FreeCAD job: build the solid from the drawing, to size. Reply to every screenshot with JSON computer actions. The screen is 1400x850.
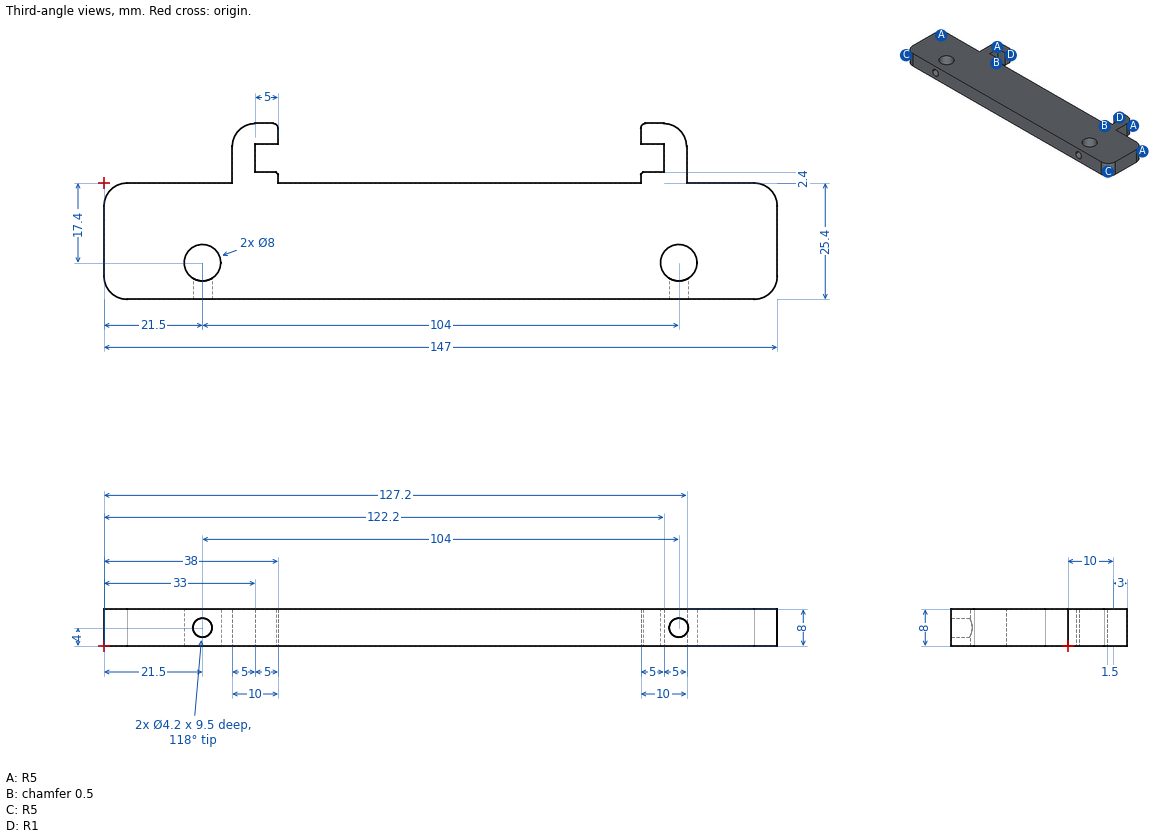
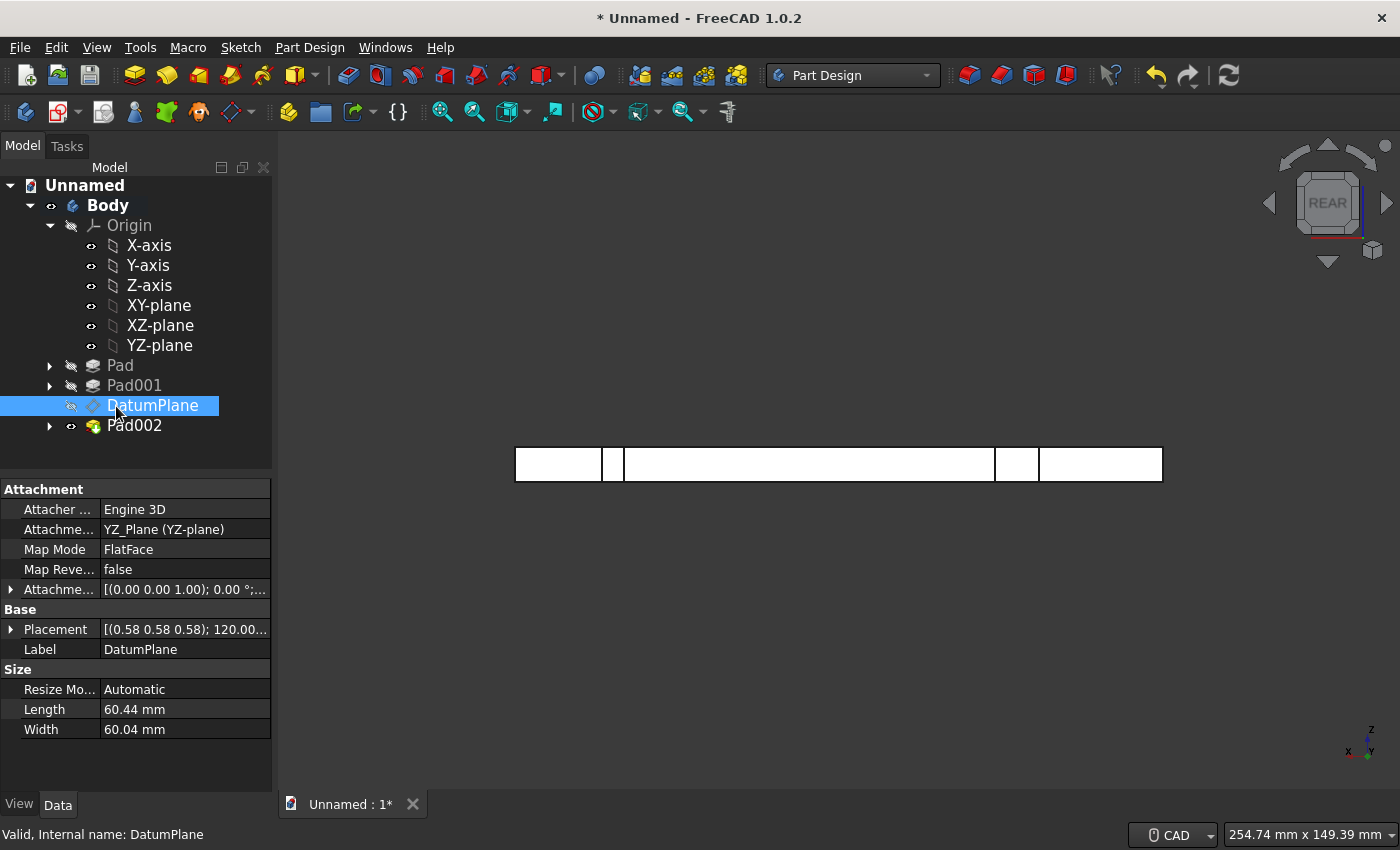
{"action": "left_click", "coordinate": [136, 346]}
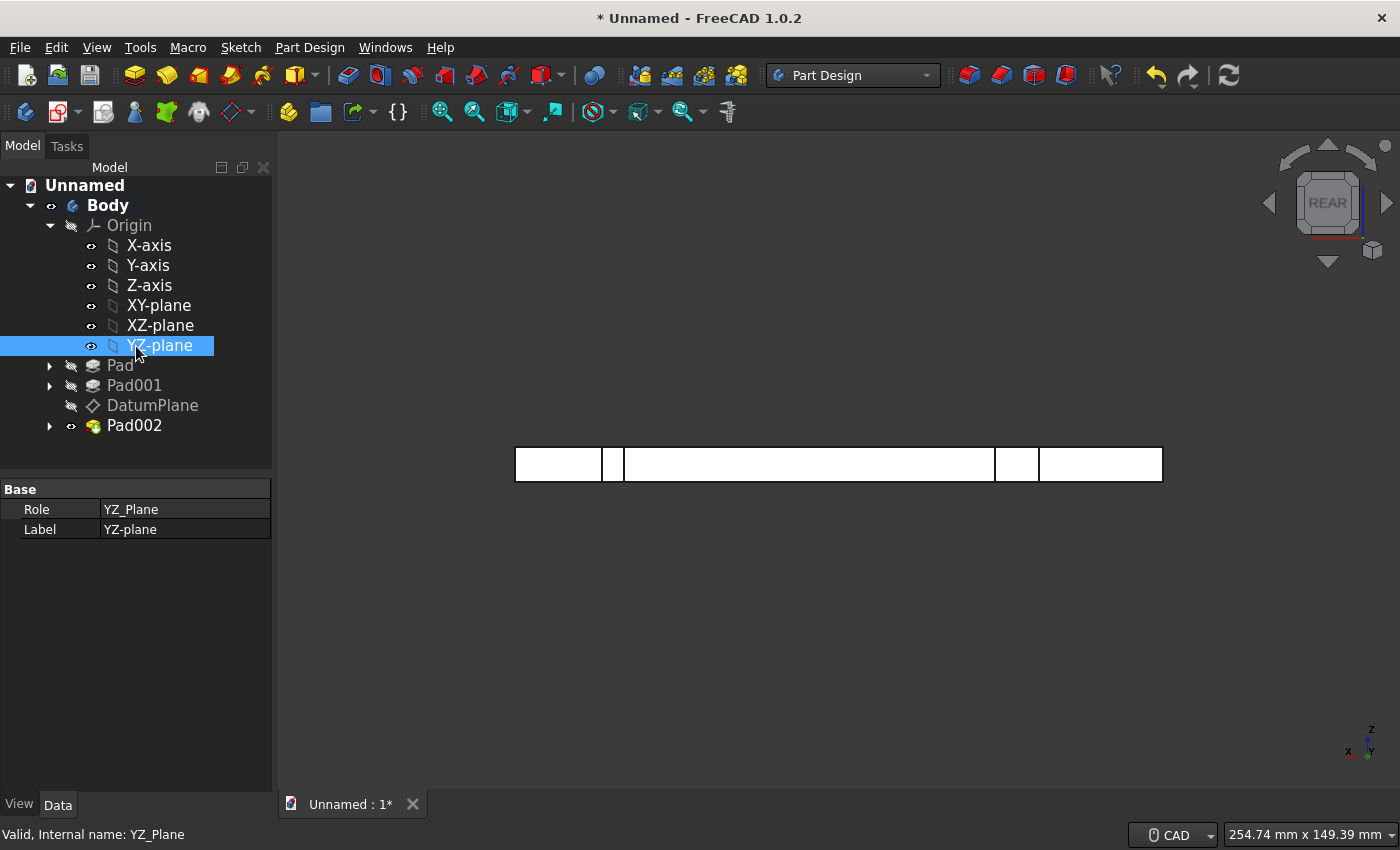
{"action": "left_click", "coordinate": [232, 112]}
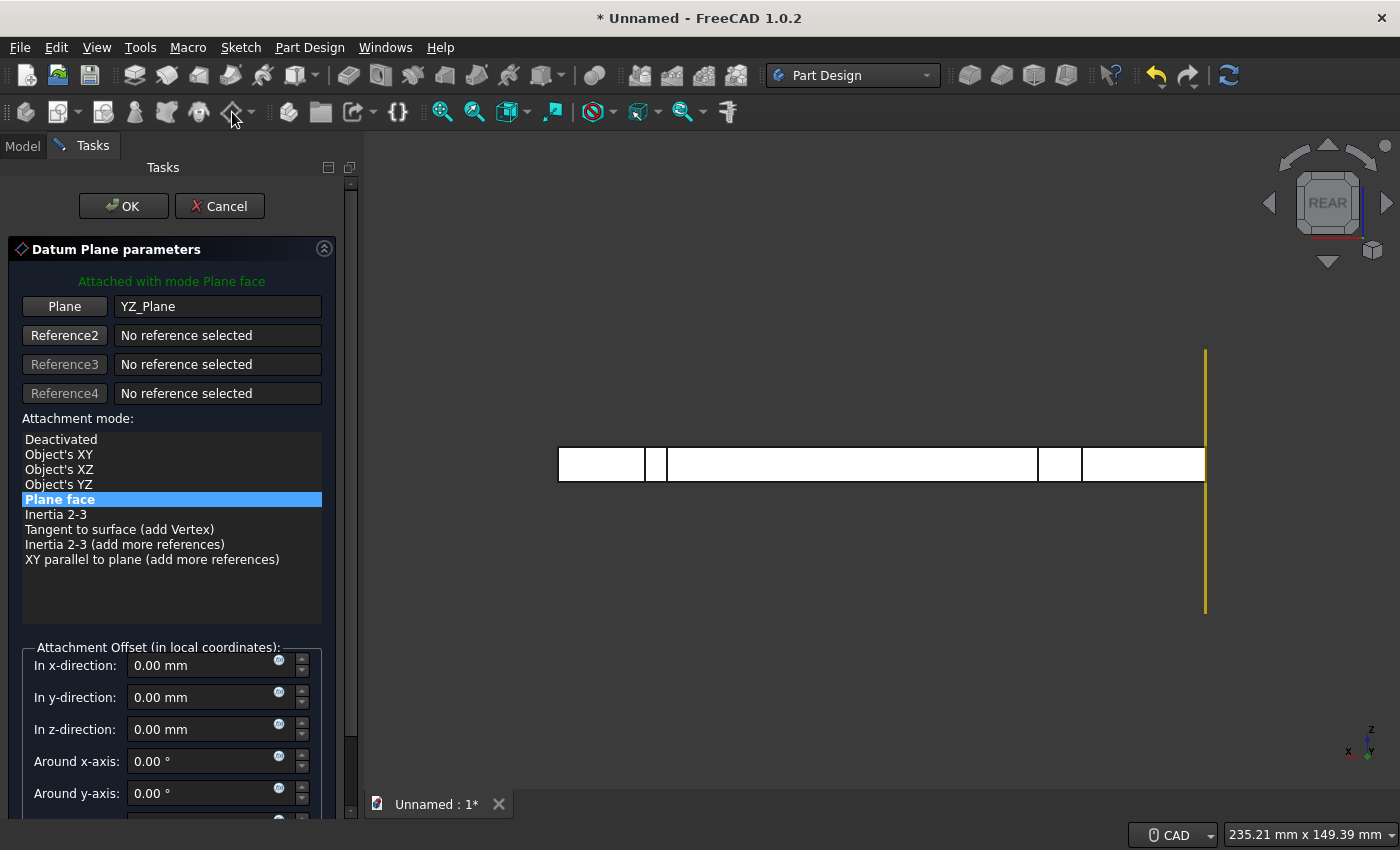
{"action": "triple_click", "coordinate": [210, 729]}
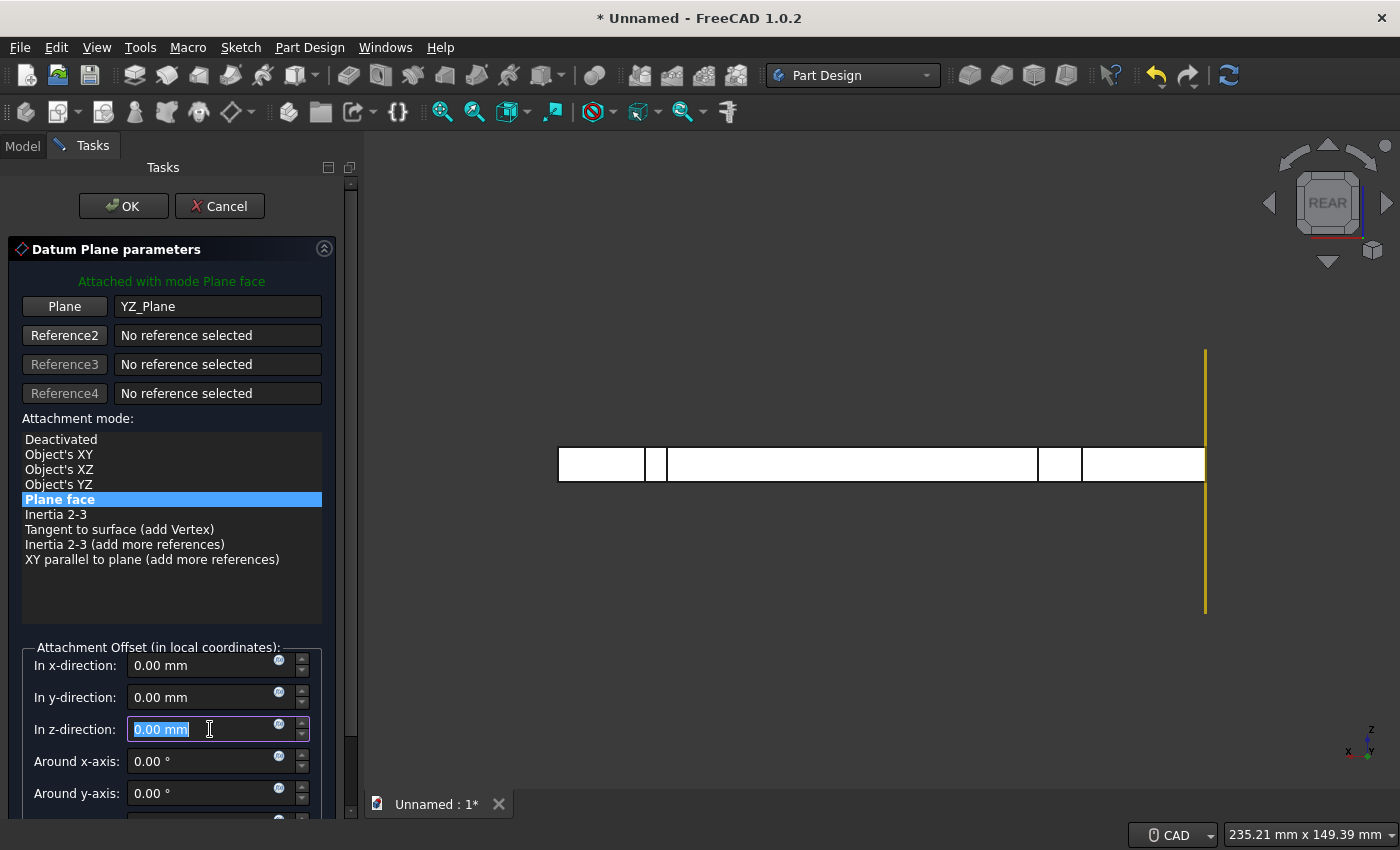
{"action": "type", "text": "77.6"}
{"action": "key", "text": "Tab"}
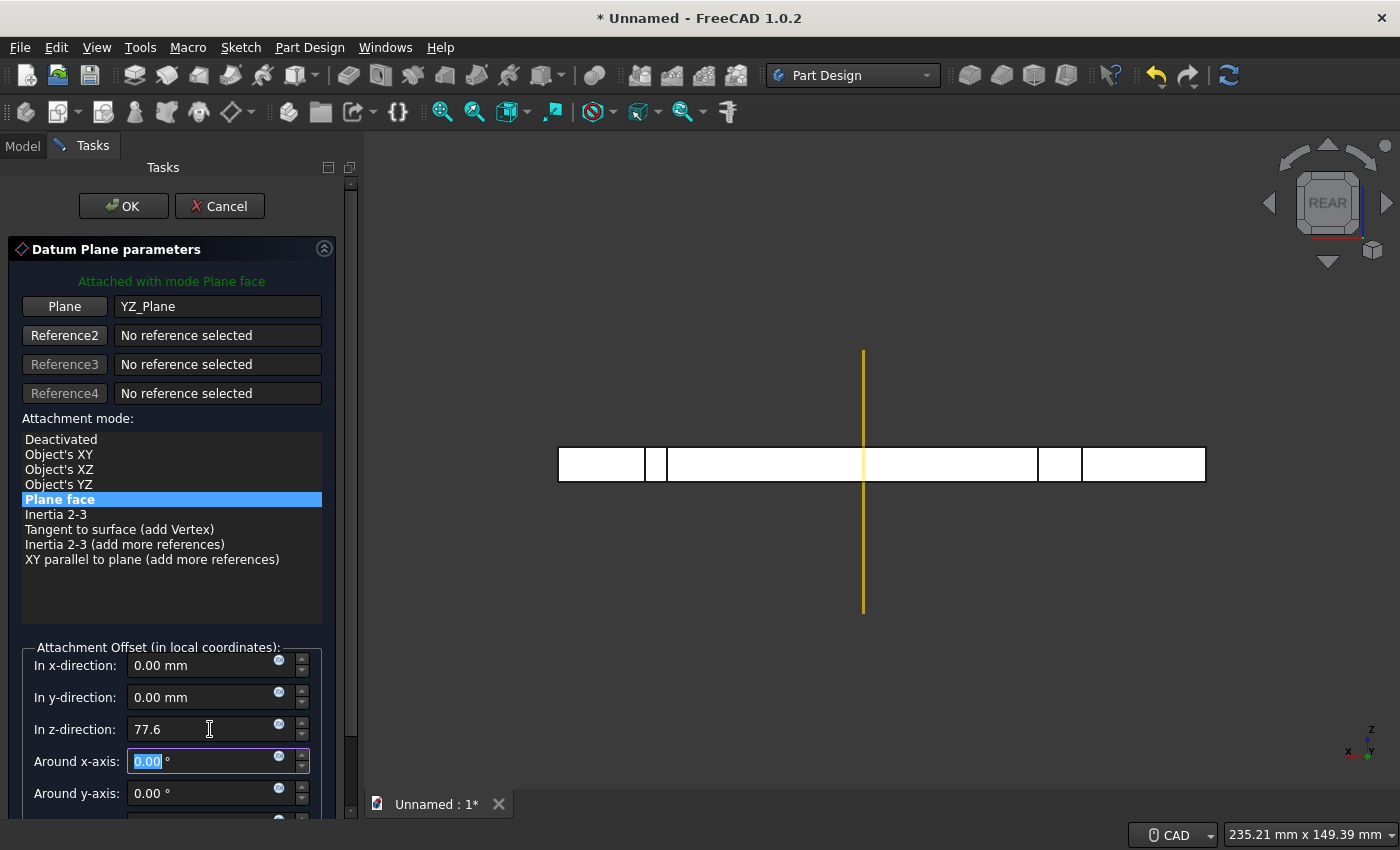
{"action": "left_click", "coordinate": [124, 206]}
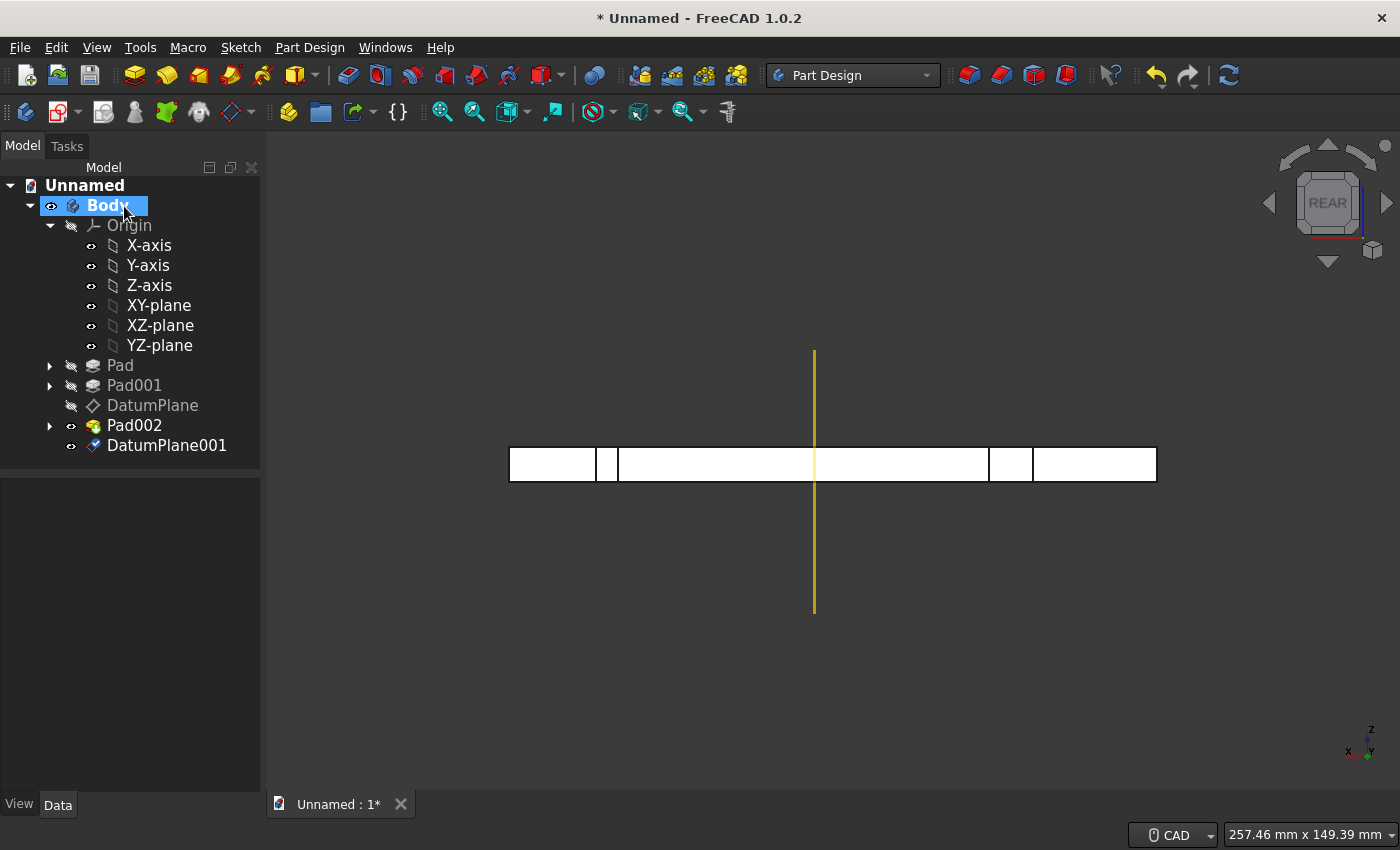
{"action": "left_click", "coordinate": [116, 426]}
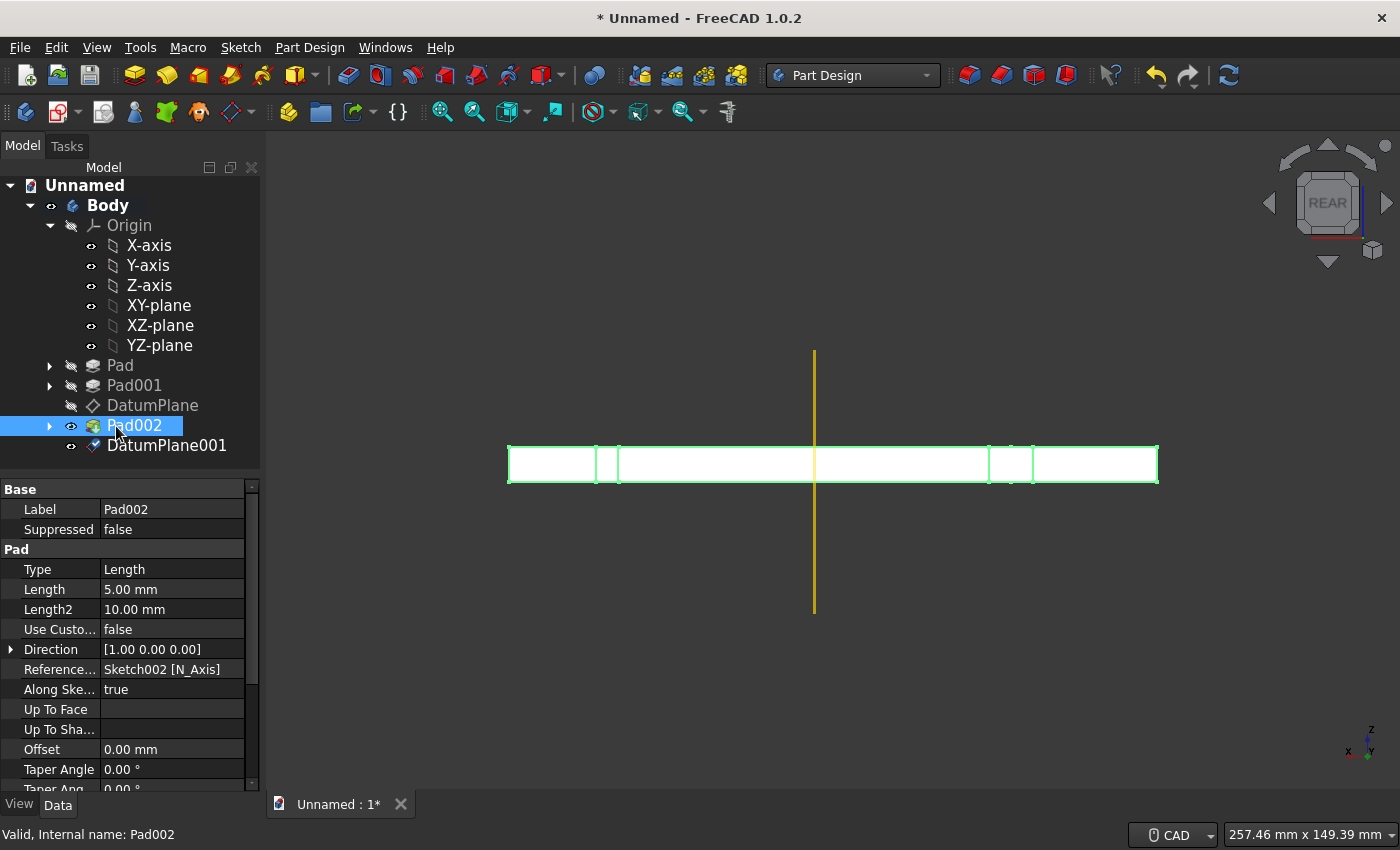
{"action": "left_click", "coordinate": [640, 76]}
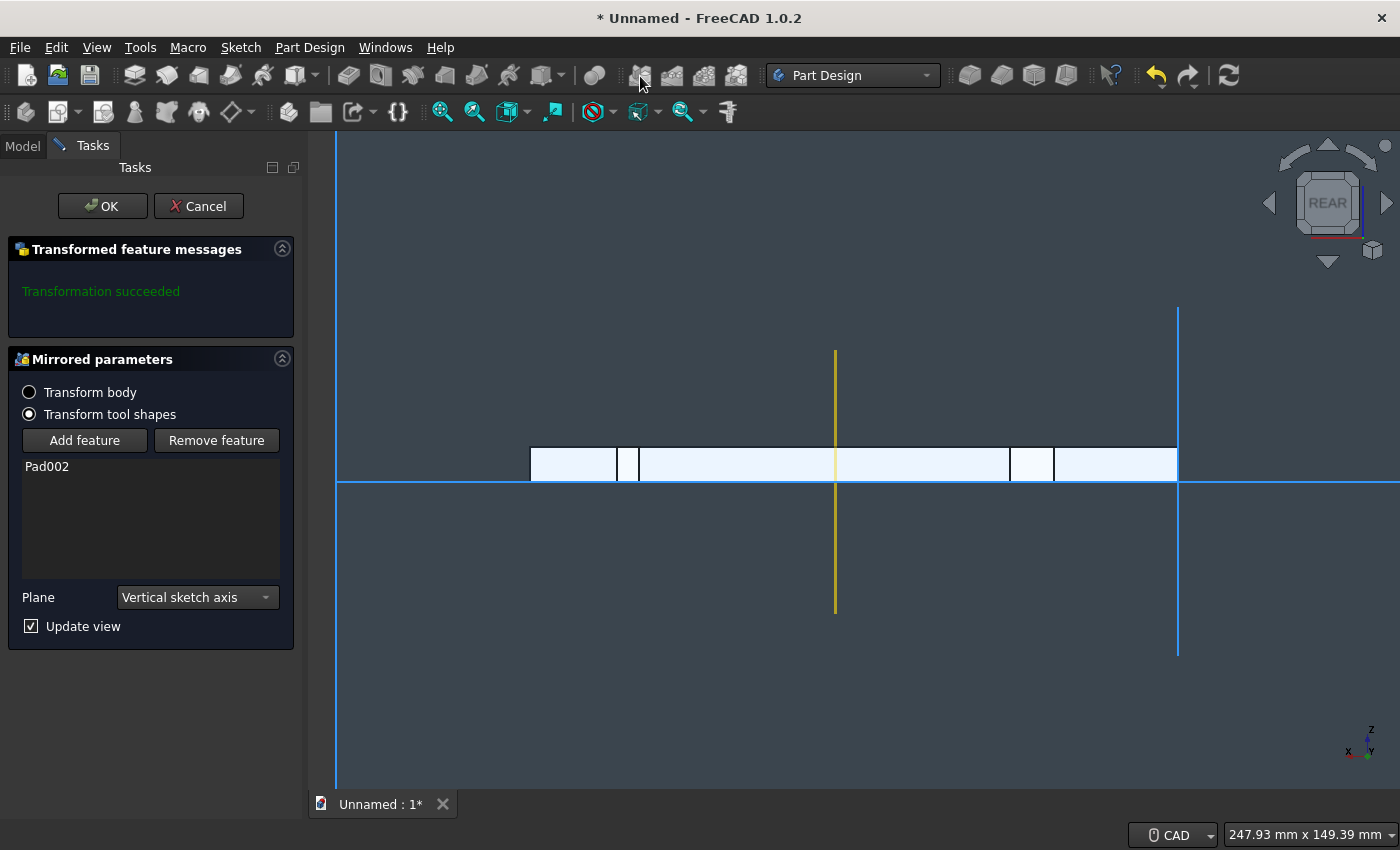
{"action": "left_click", "coordinate": [198, 598]}